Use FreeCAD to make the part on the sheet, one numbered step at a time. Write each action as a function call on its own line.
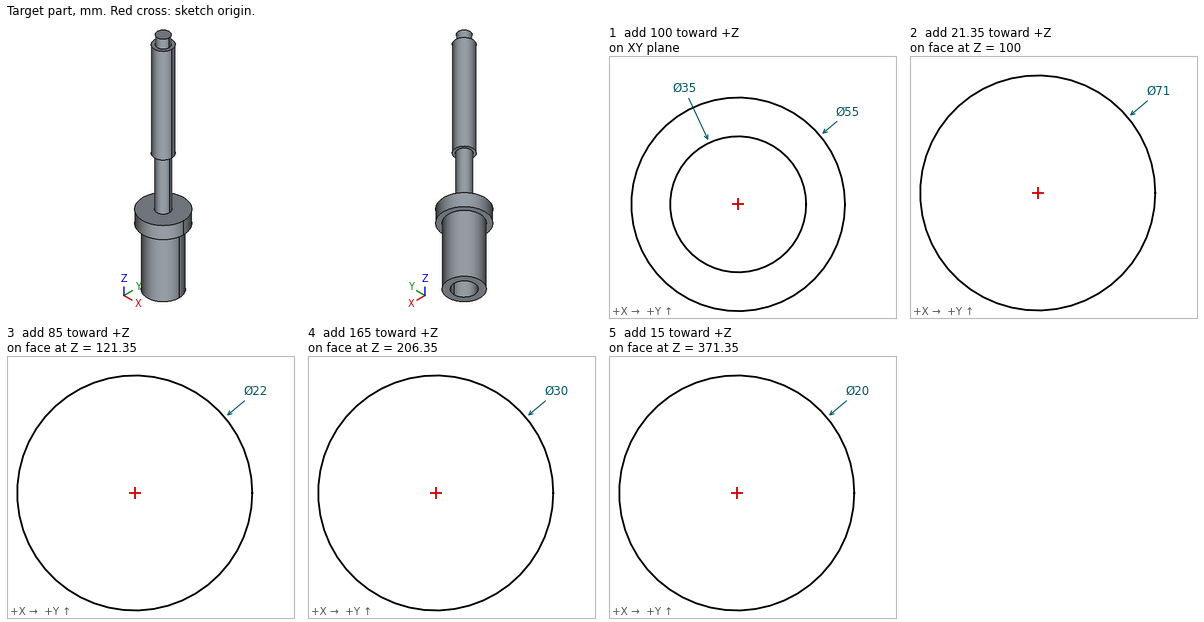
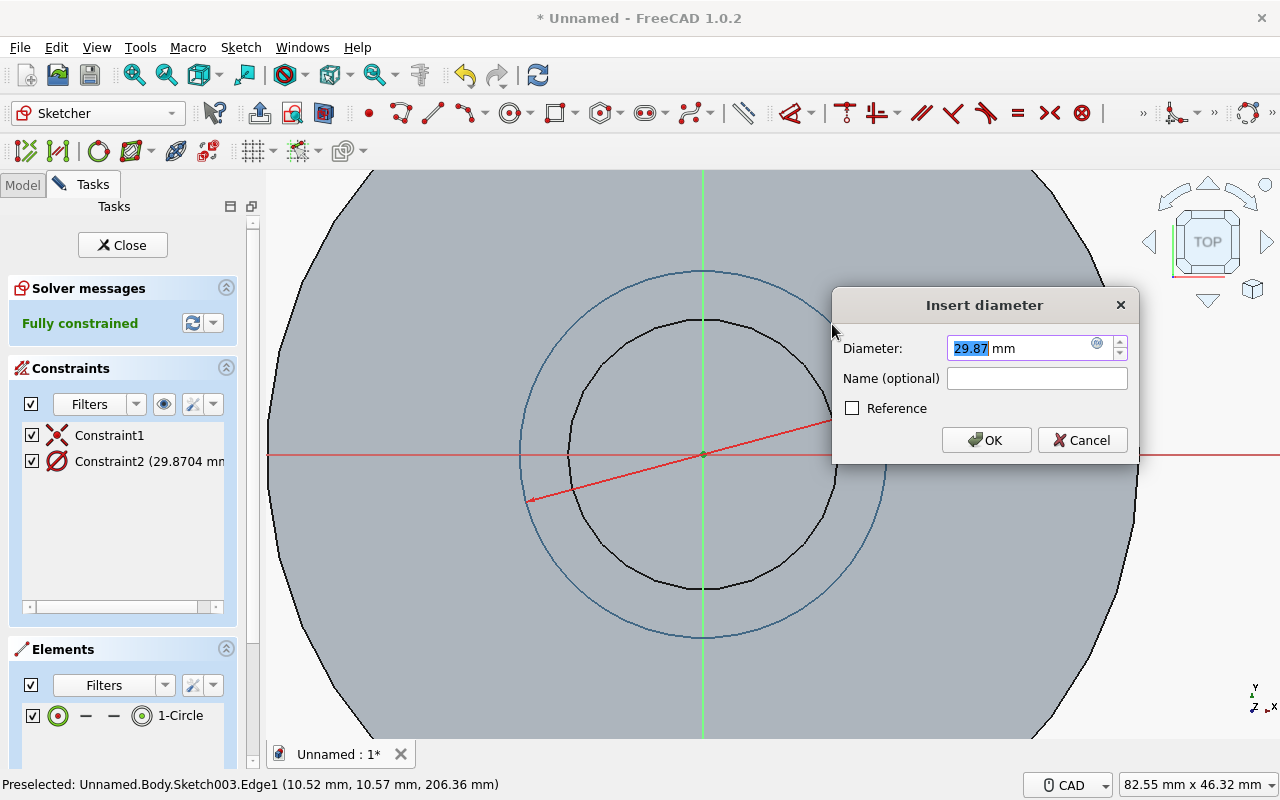
text(30)
key(Return)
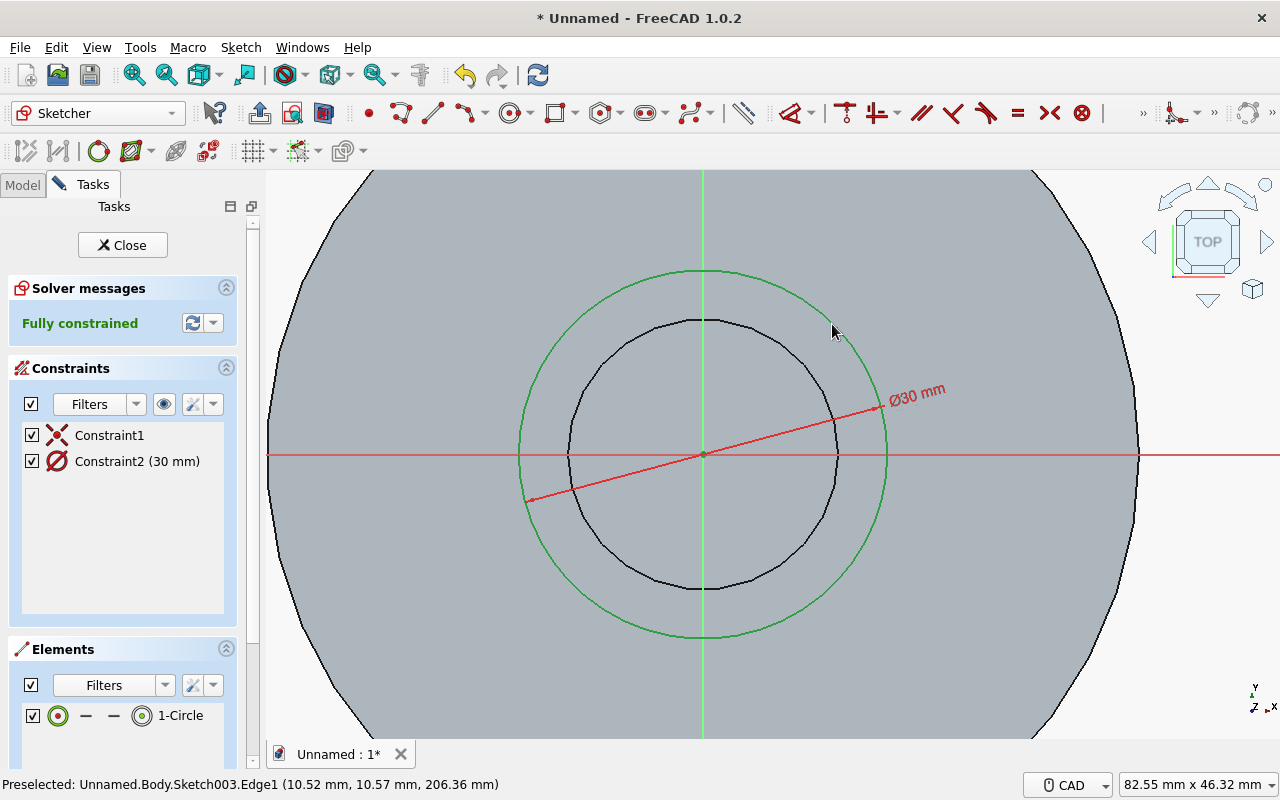
click(123, 245)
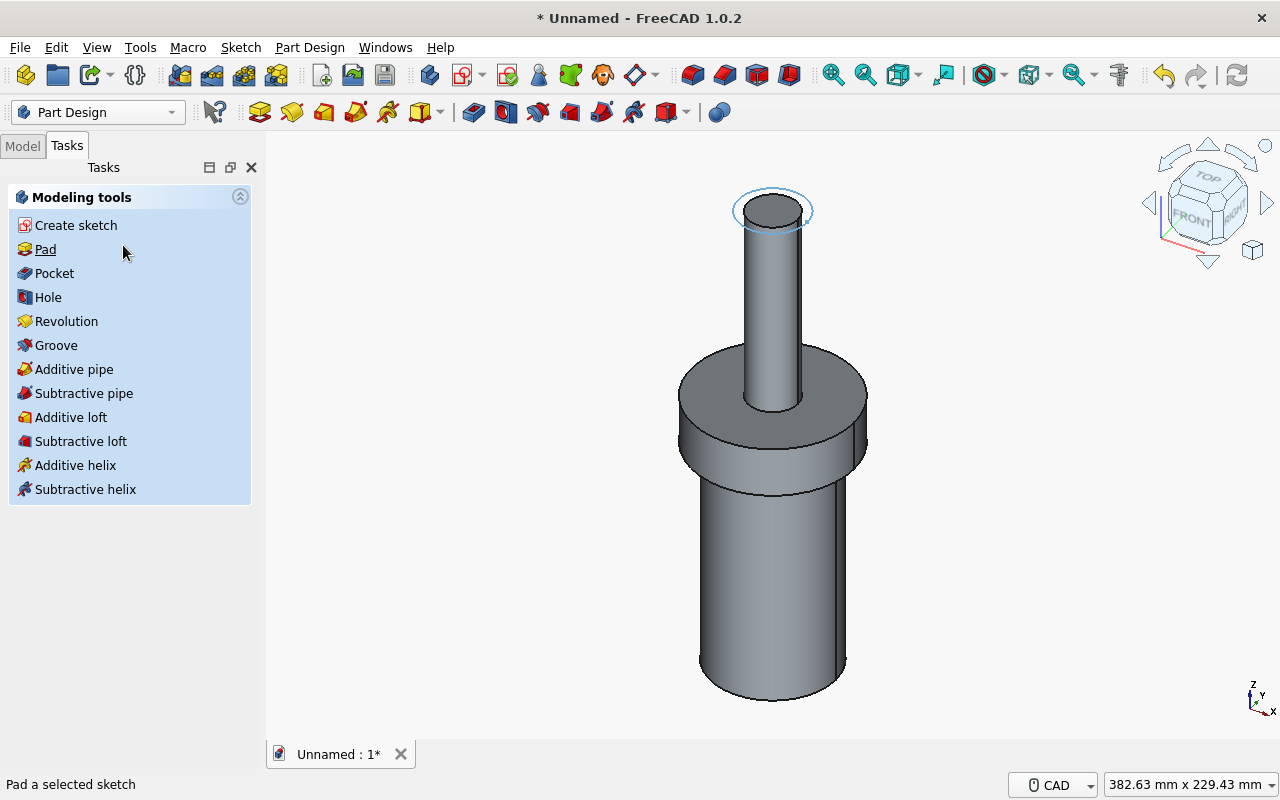
click(260, 112)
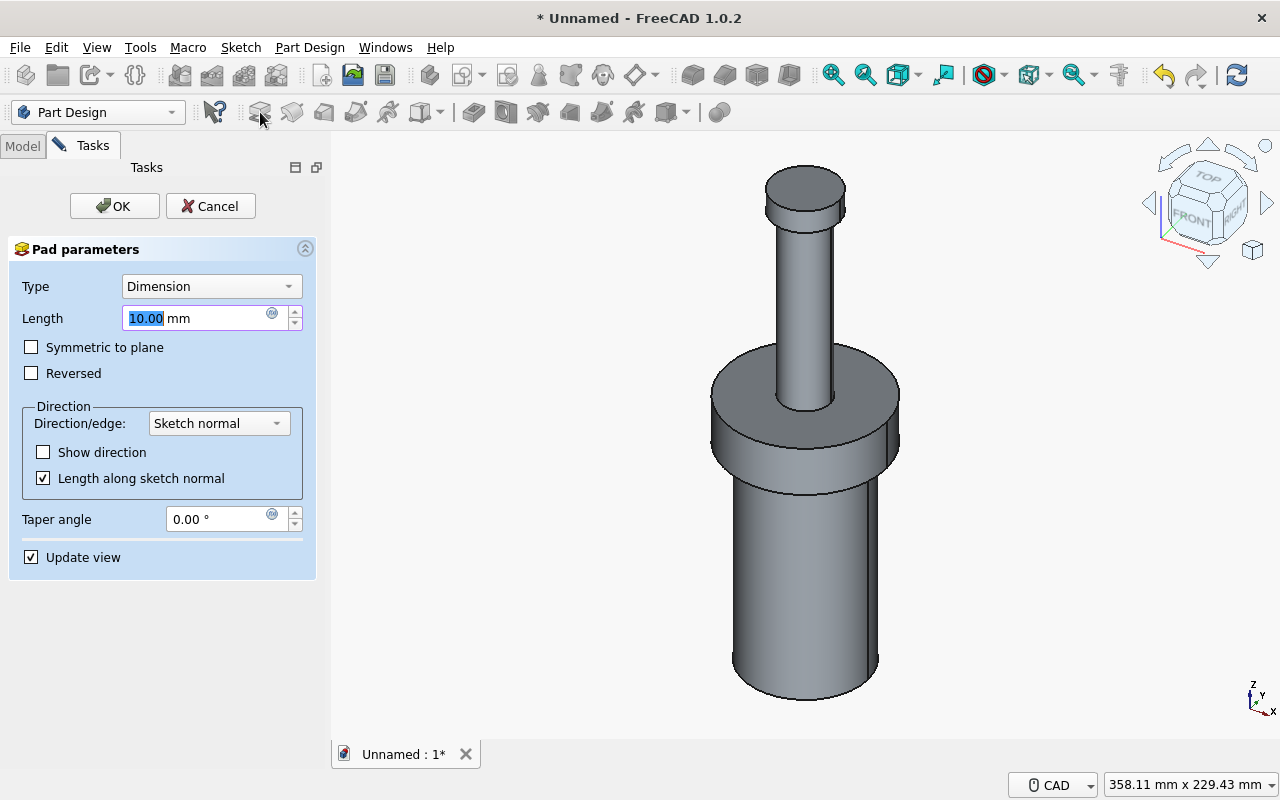
text(165)
key(Tab)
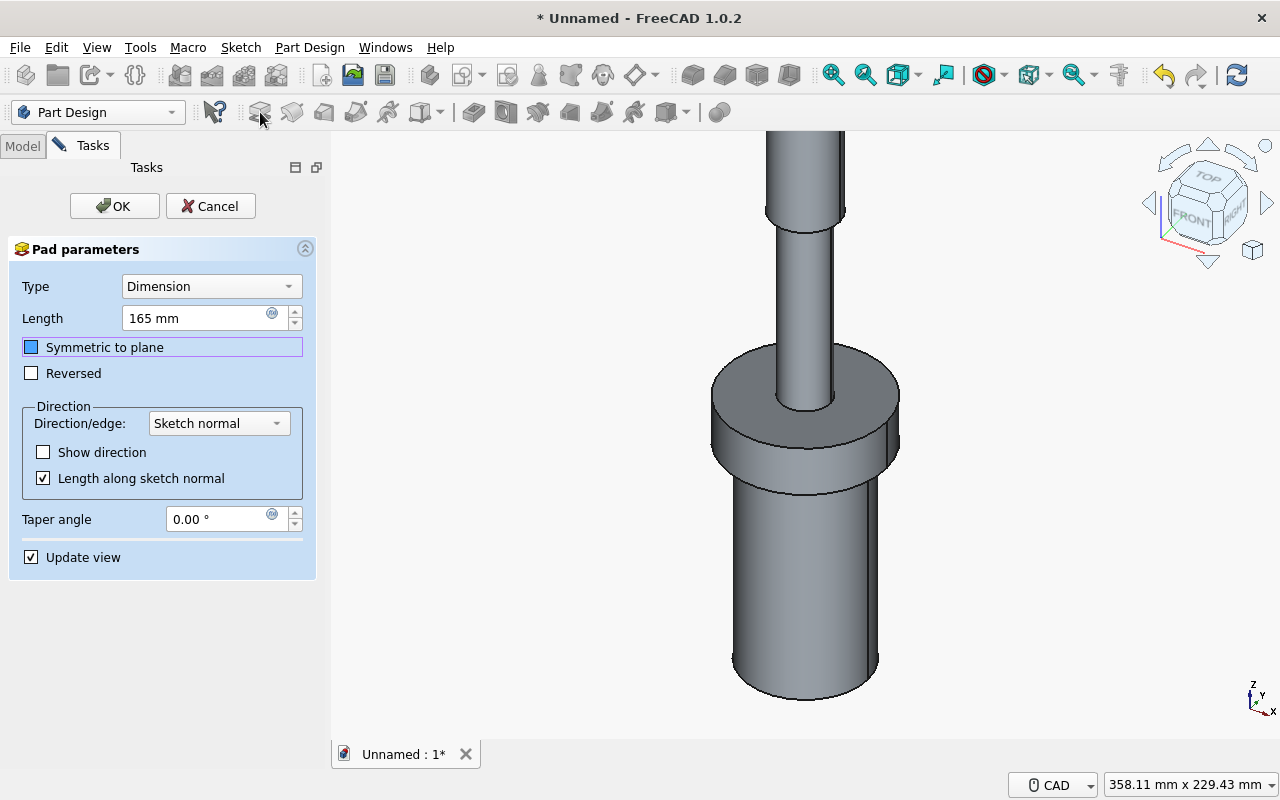
click(115, 206)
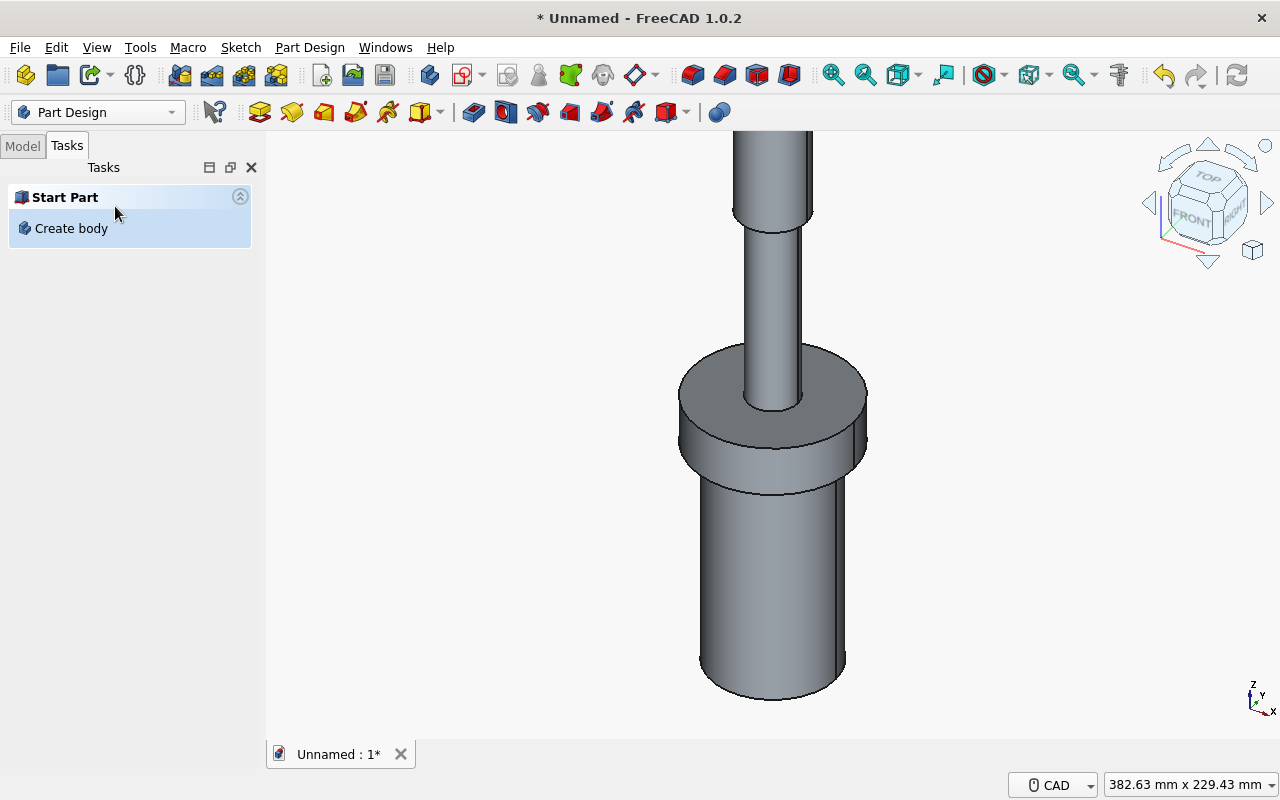
key(v)
key(f)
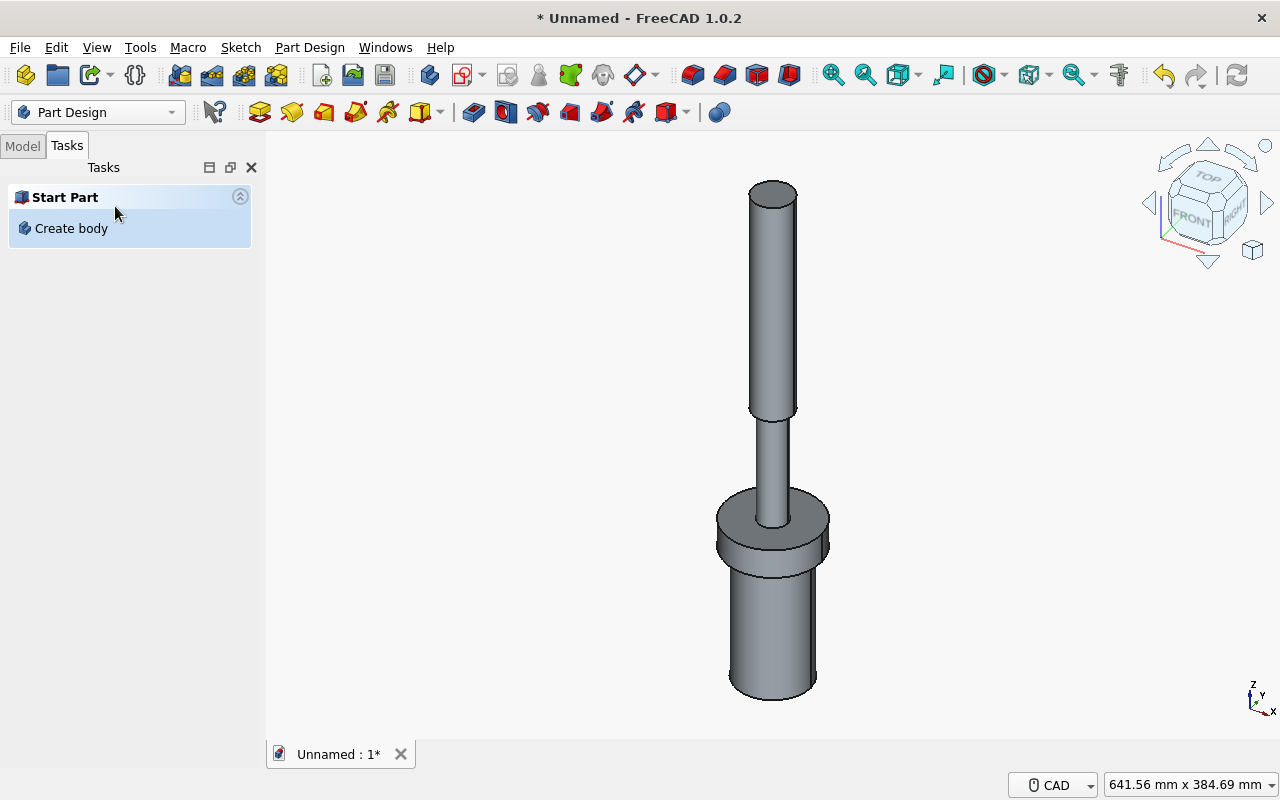
click(773, 194)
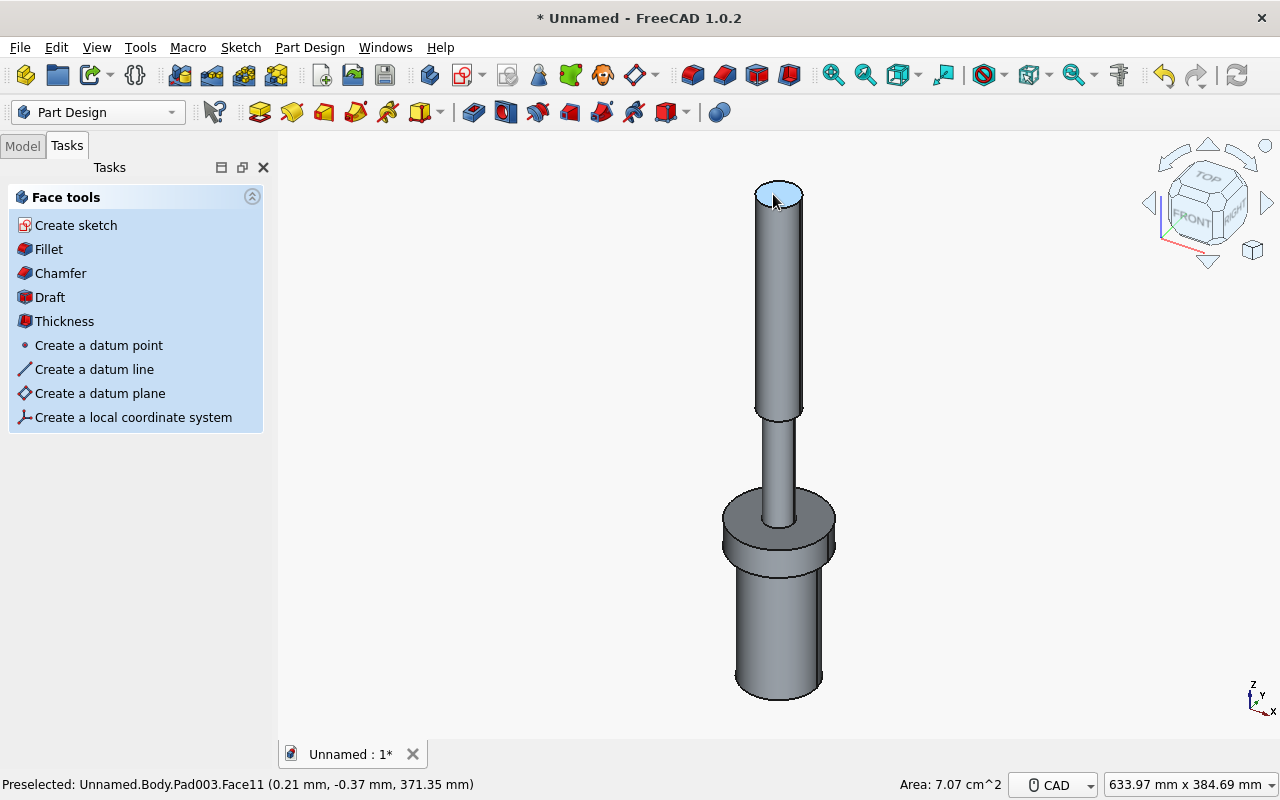
click(462, 76)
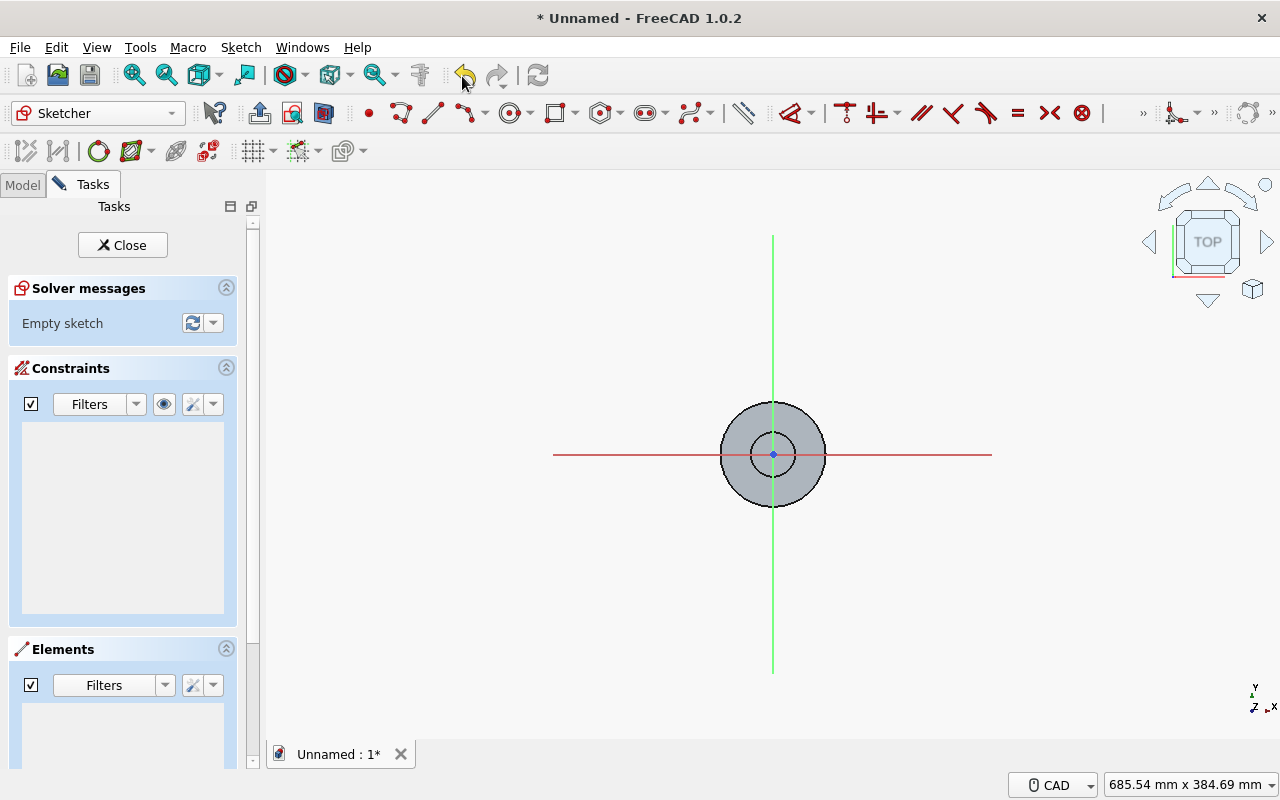
scroll(778, 454, up, 13)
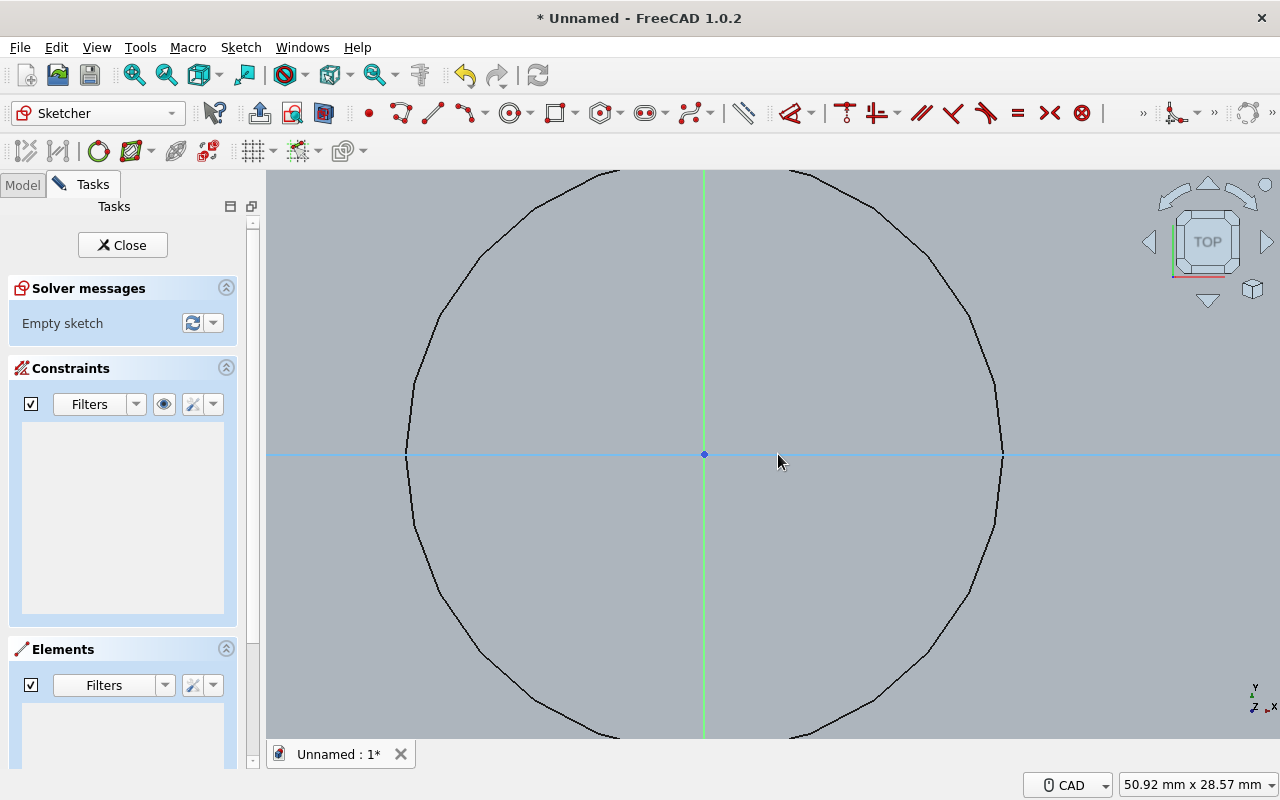
key(g)
key(c)